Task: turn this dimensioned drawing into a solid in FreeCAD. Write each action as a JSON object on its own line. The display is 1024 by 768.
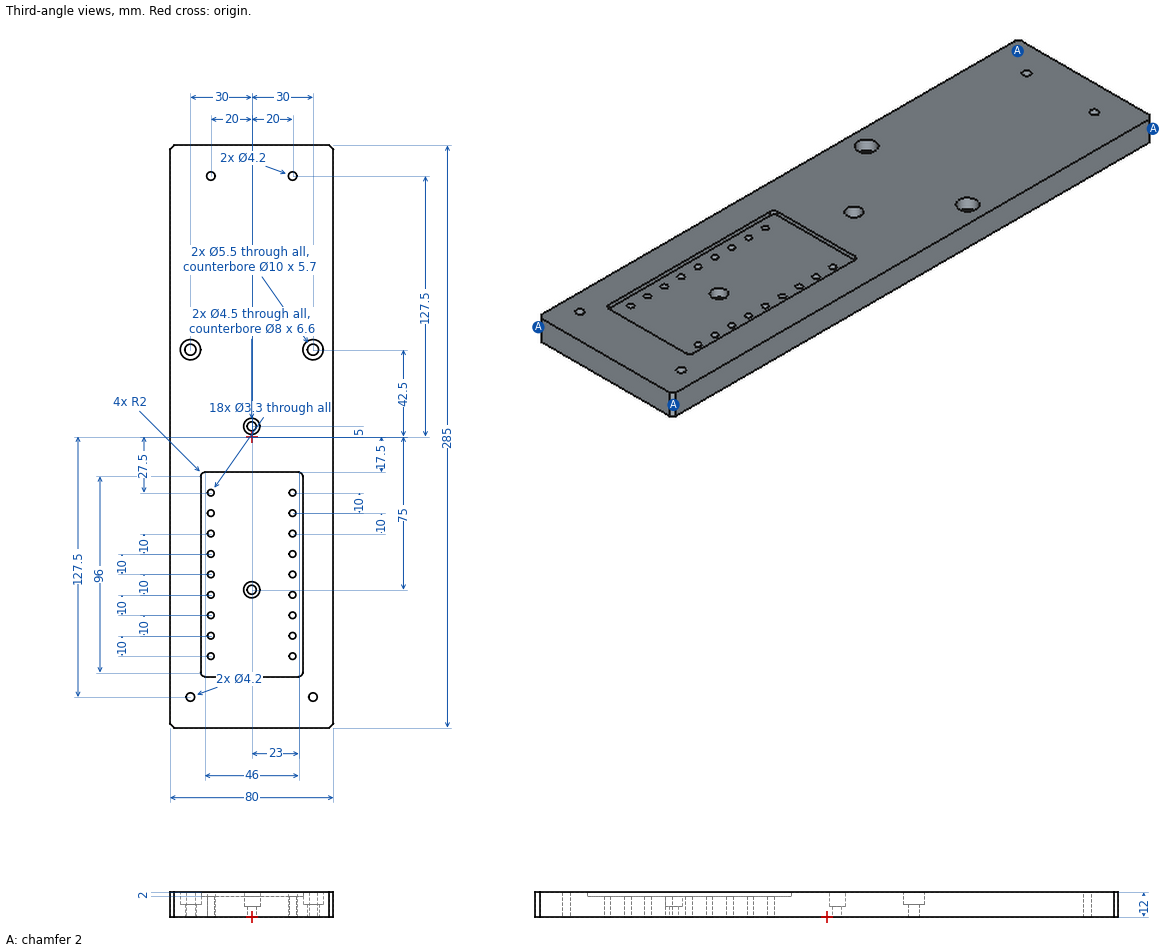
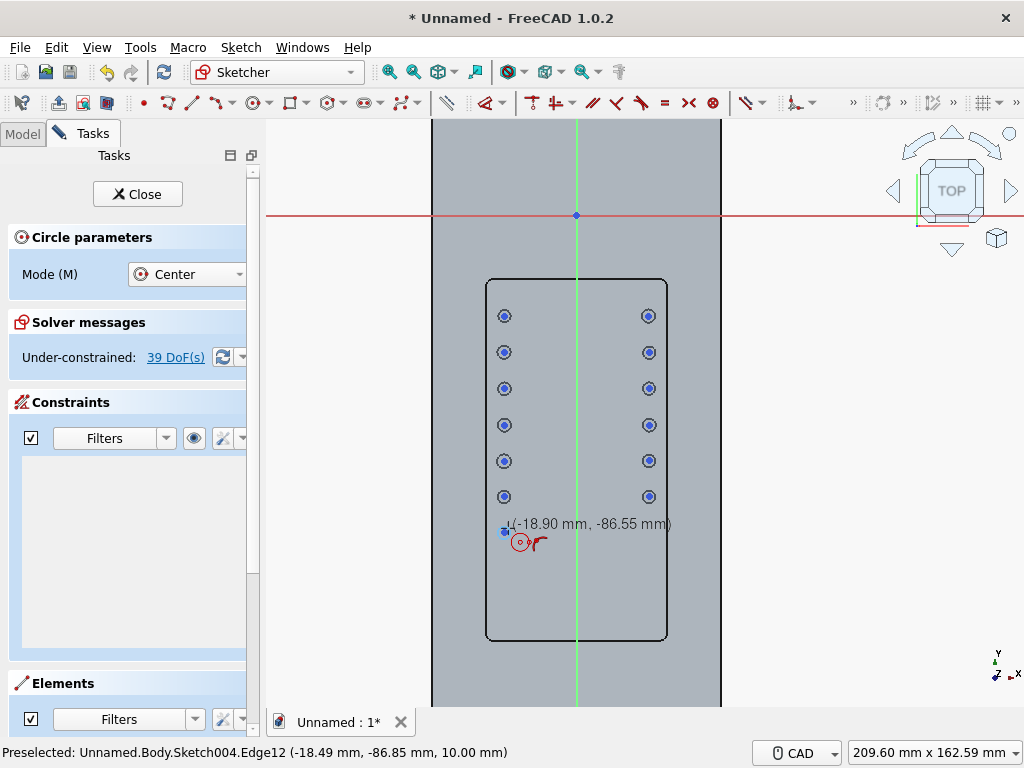
{"action": "scroll", "coordinate": [649, 532], "scroll_direction": "up", "scroll_amount": 7}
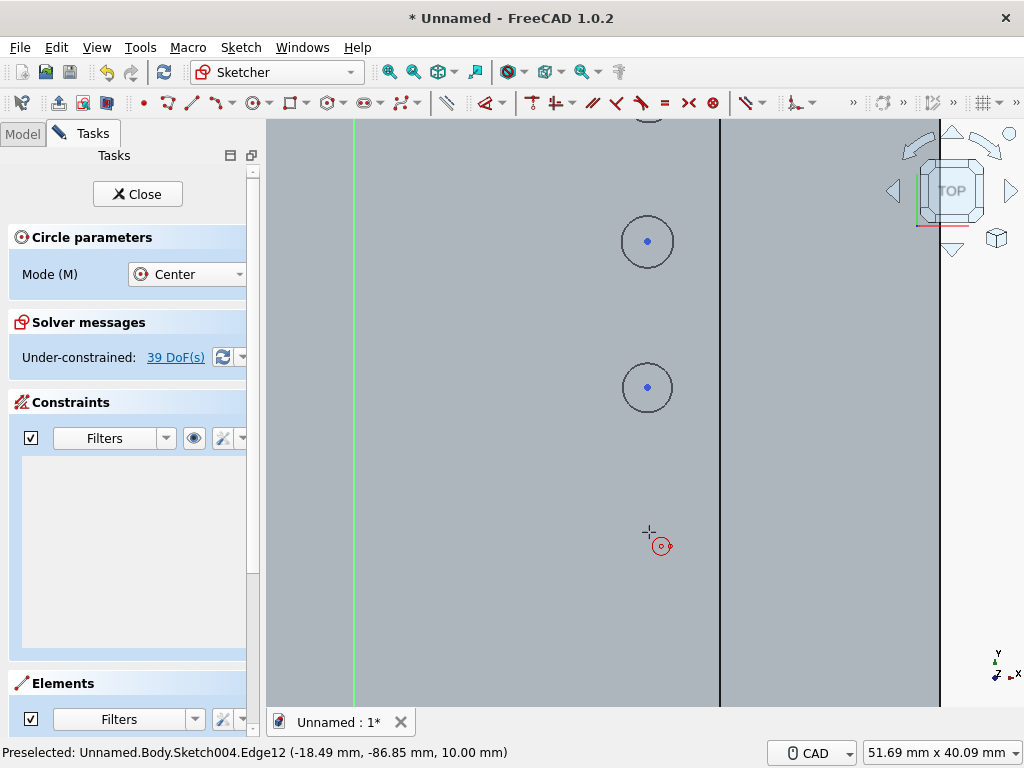
{"action": "scroll", "coordinate": [649, 532], "scroll_direction": "down", "scroll_amount": 7}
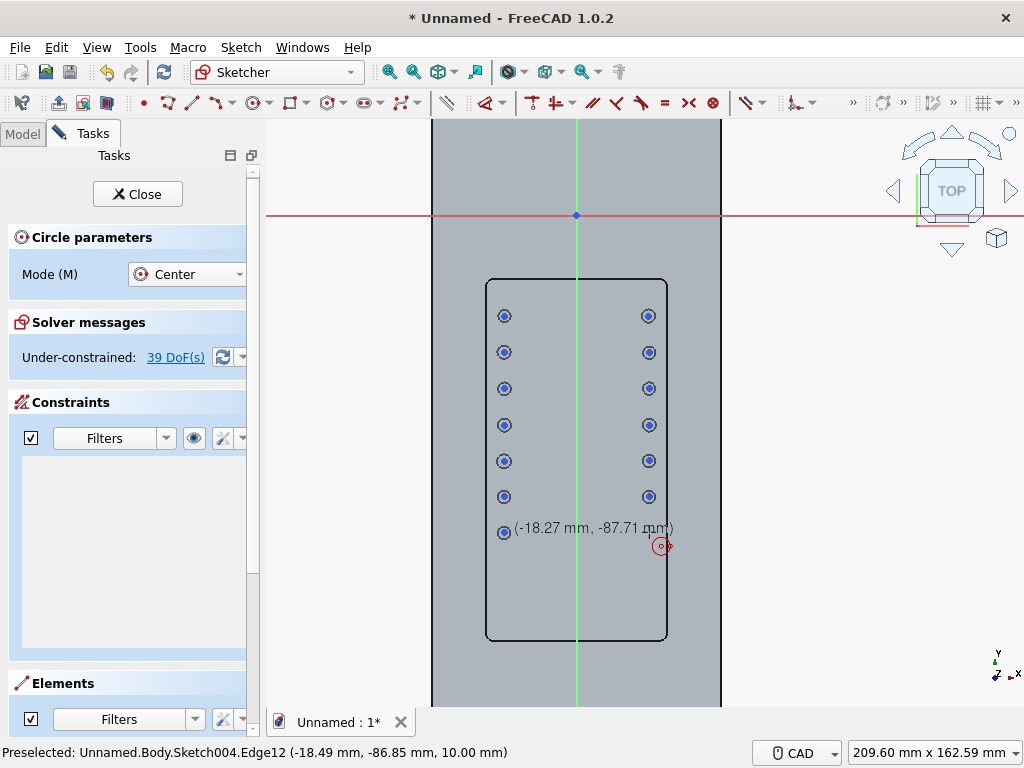
{"action": "left_click", "coordinate": [649, 532]}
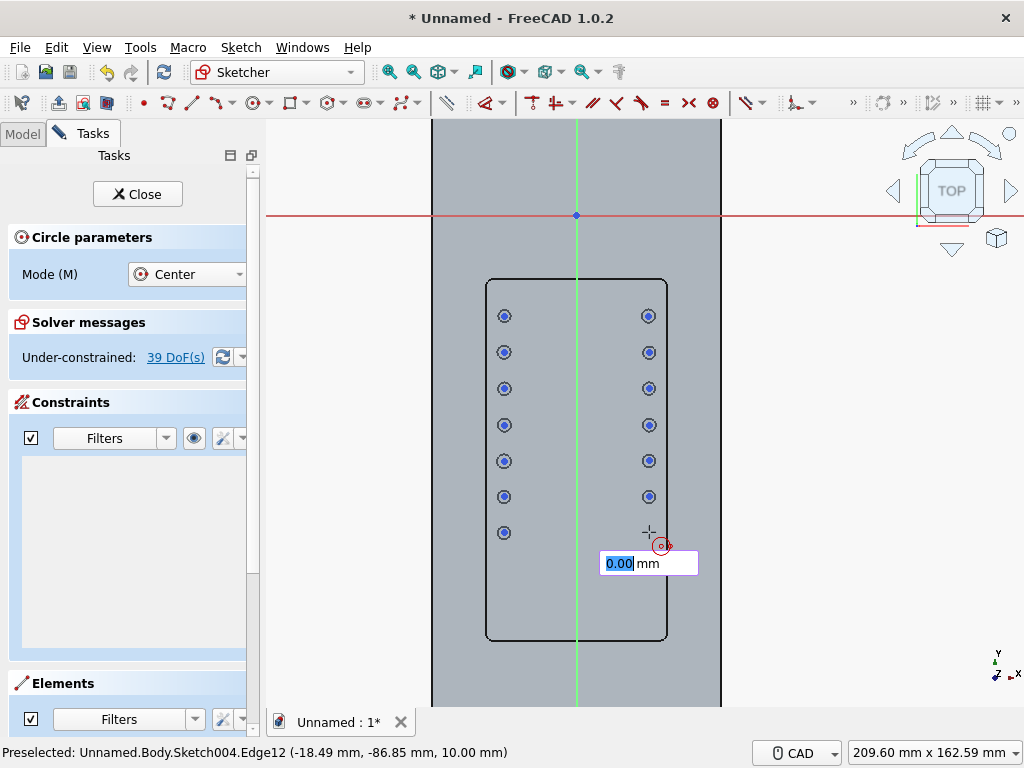
{"action": "scroll", "coordinate": [653, 528], "scroll_direction": "up", "scroll_amount": 5}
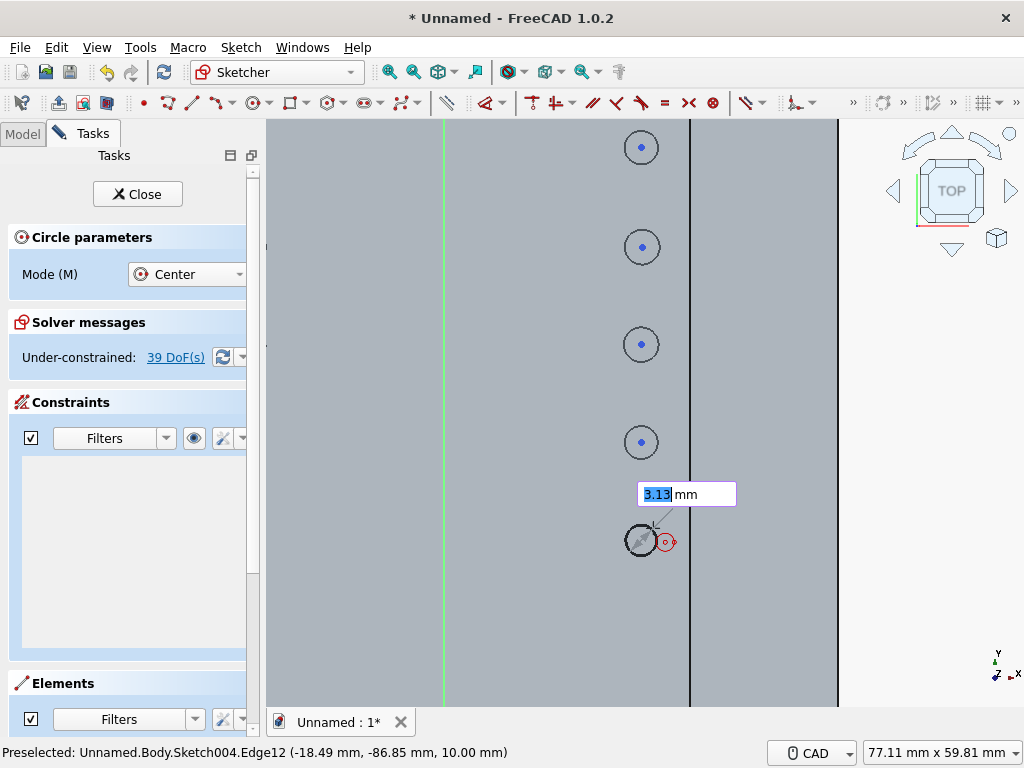
{"action": "left_click", "coordinate": [652, 527]}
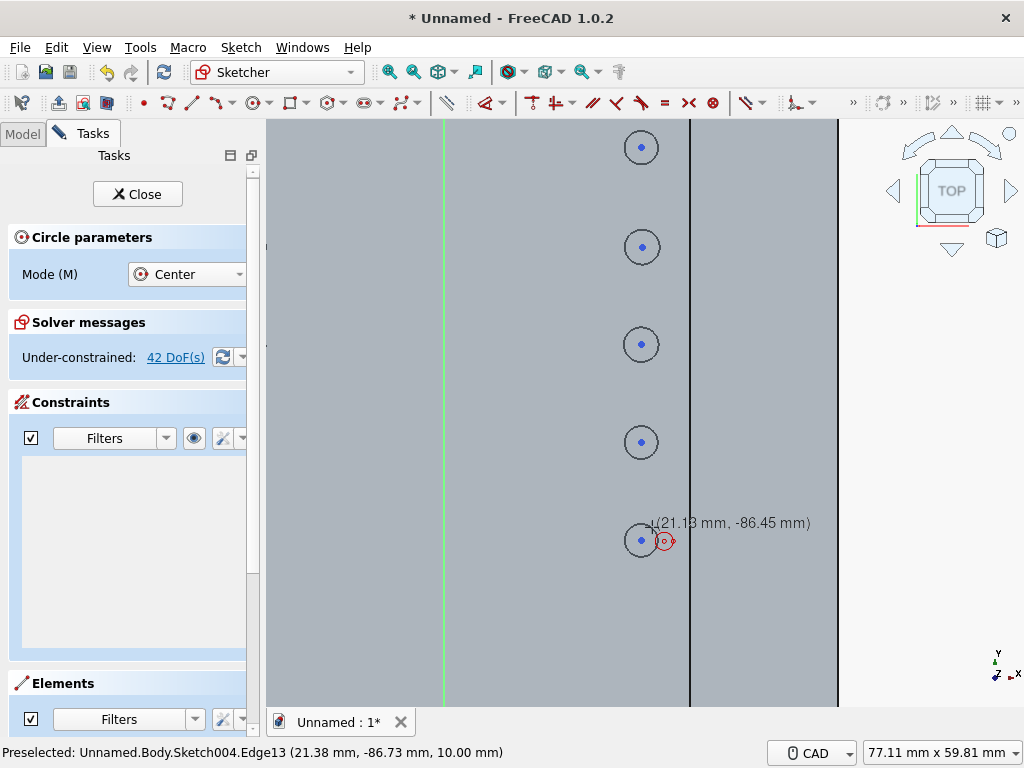
{"action": "scroll", "coordinate": [653, 528], "scroll_direction": "down", "scroll_amount": 5}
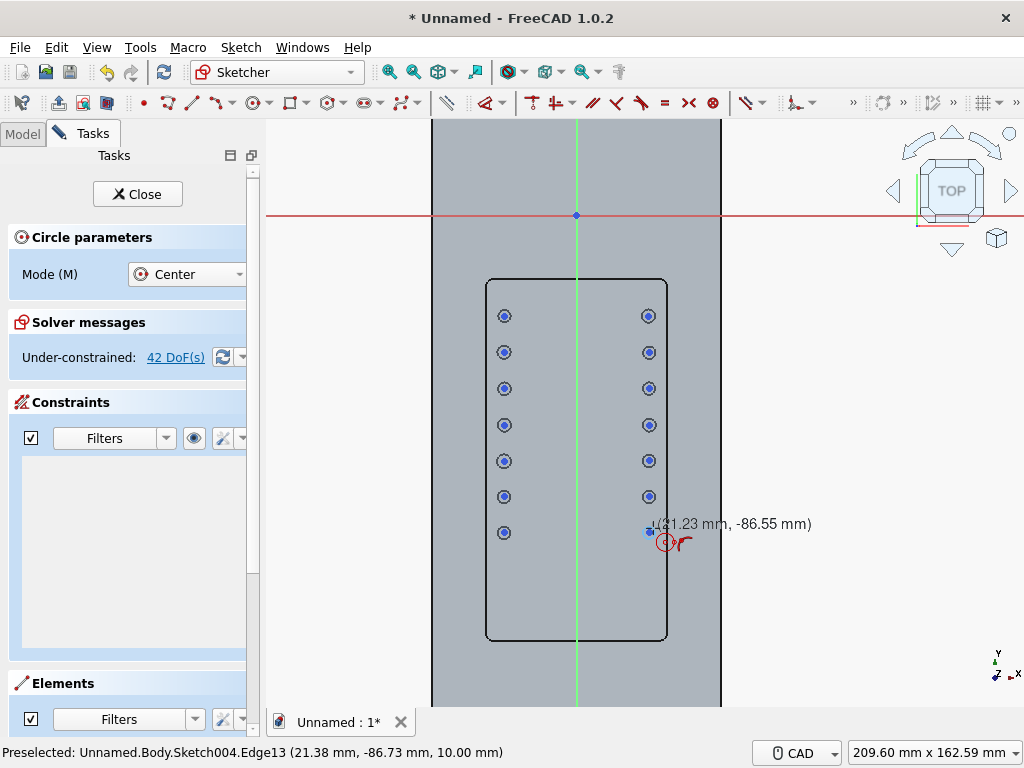
{"action": "scroll", "coordinate": [504, 568], "scroll_direction": "up", "scroll_amount": 7}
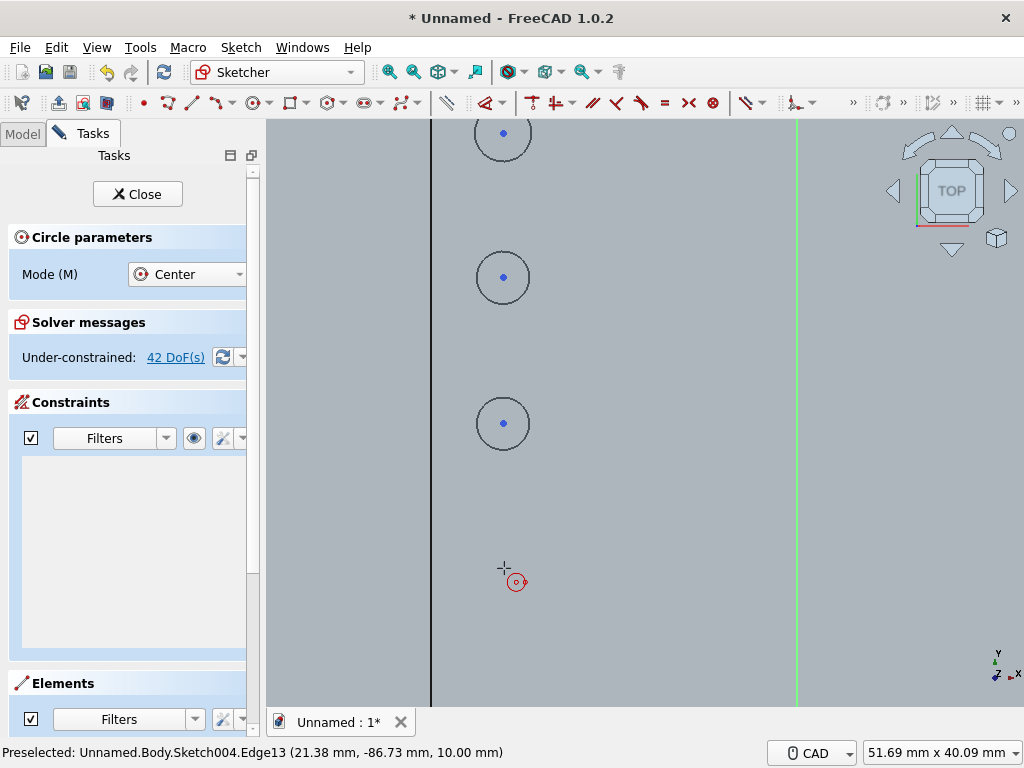
{"action": "scroll", "coordinate": [504, 569], "scroll_direction": "down", "scroll_amount": 7}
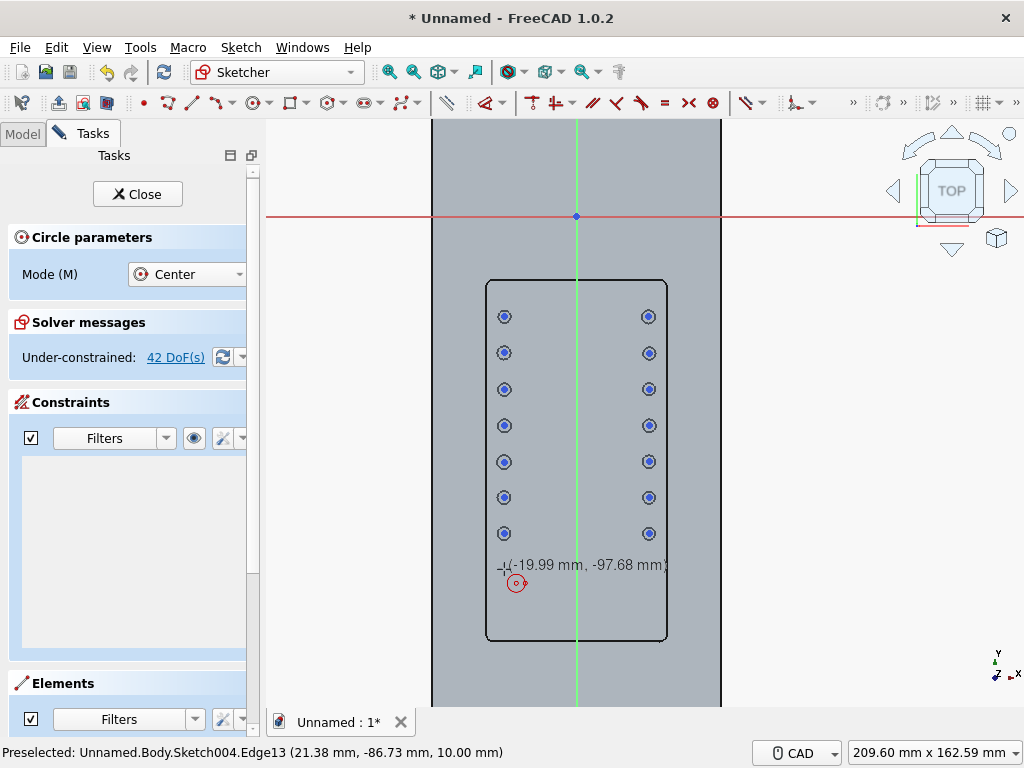
{"action": "left_click", "coordinate": [504, 569]}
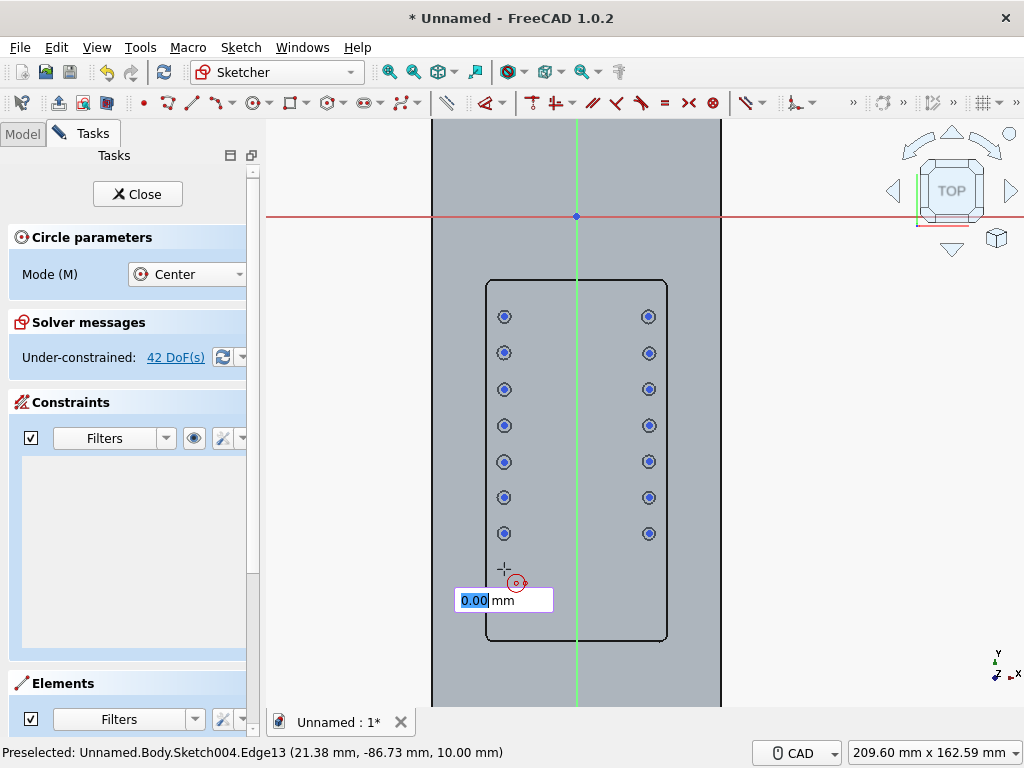
{"action": "scroll", "coordinate": [508, 565], "scroll_direction": "up", "scroll_amount": 5}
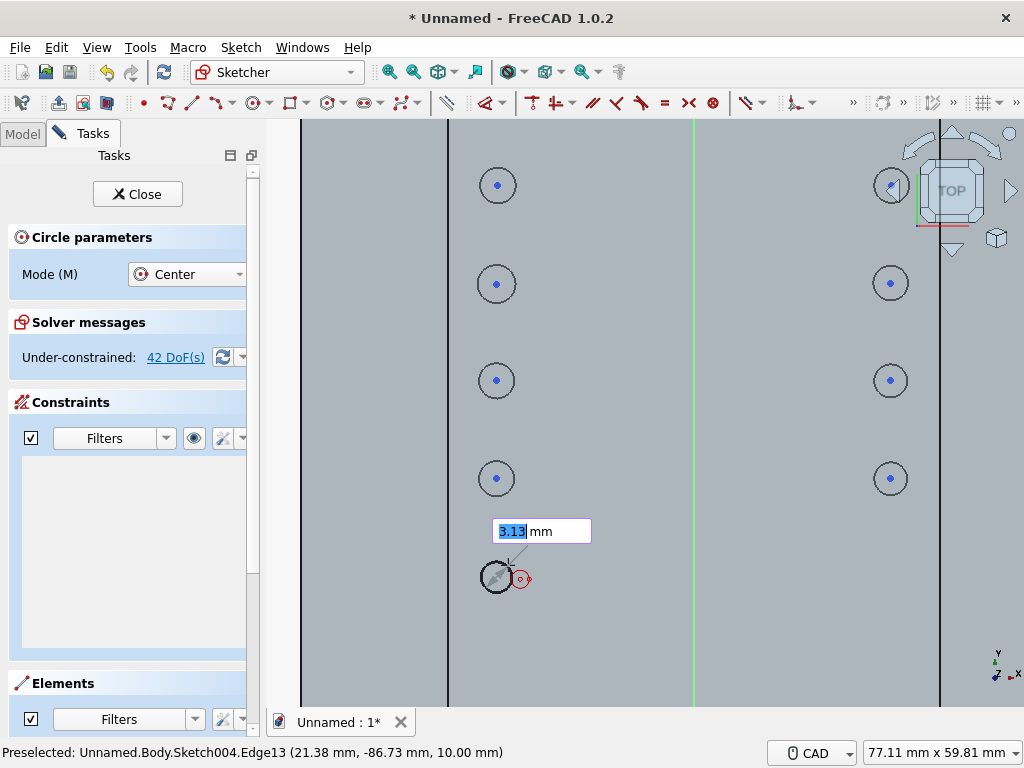
{"action": "left_click", "coordinate": [509, 564]}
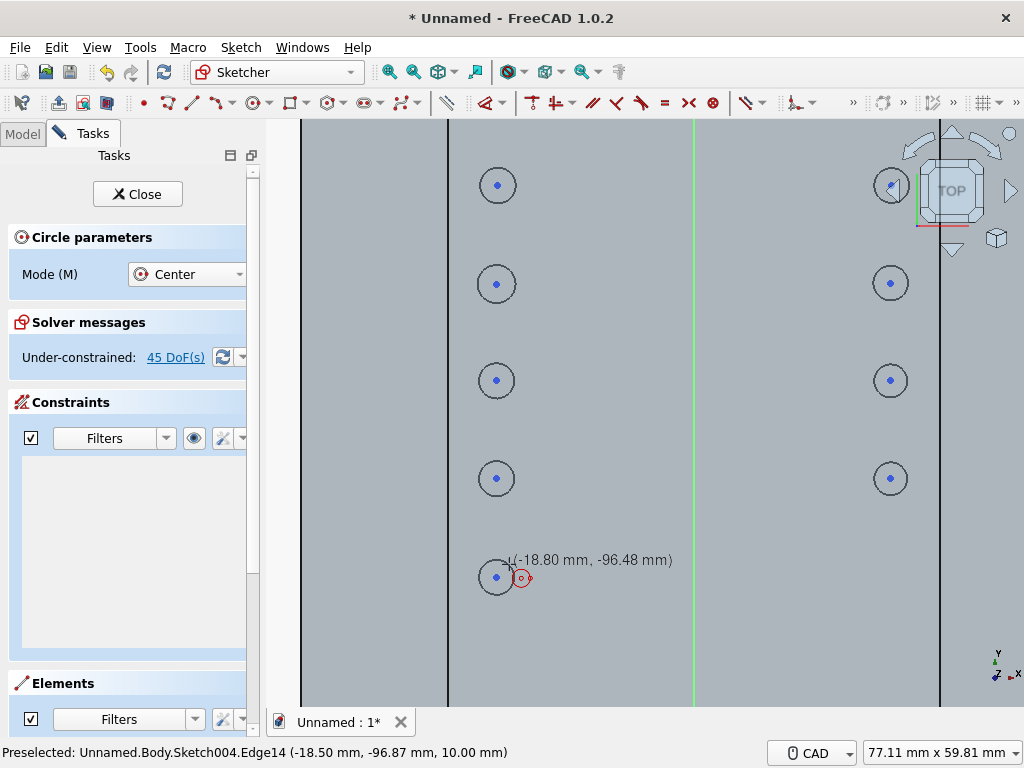
{"action": "scroll", "coordinate": [508, 564], "scroll_direction": "down", "scroll_amount": 5}